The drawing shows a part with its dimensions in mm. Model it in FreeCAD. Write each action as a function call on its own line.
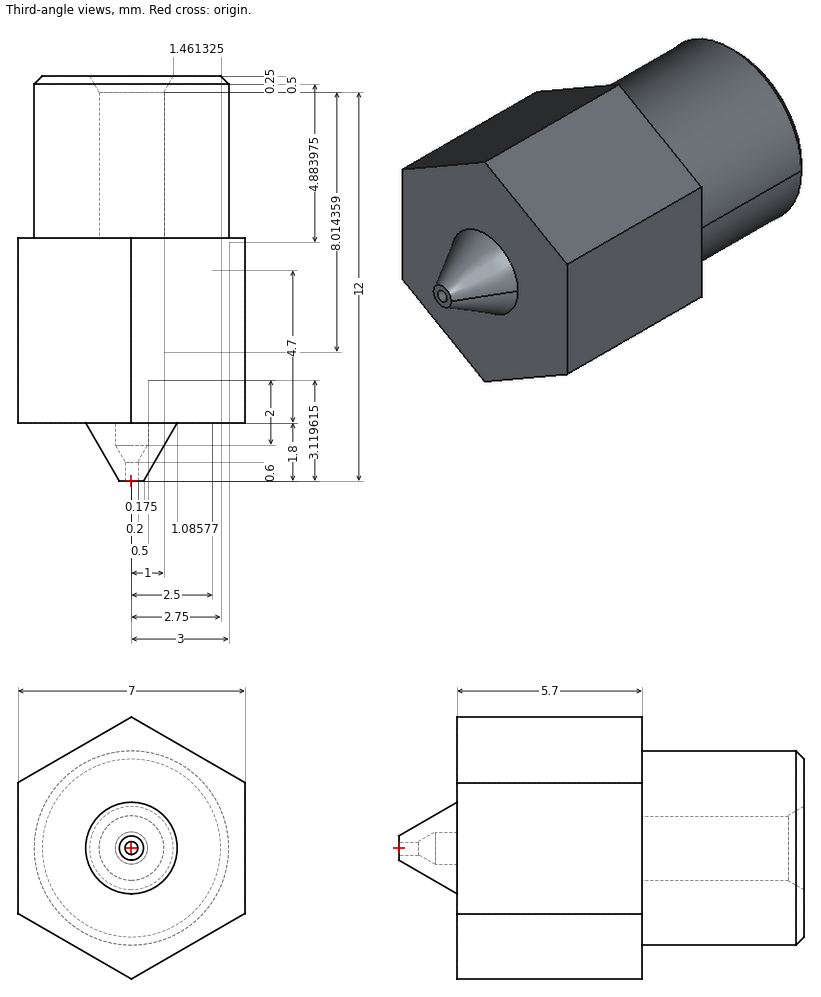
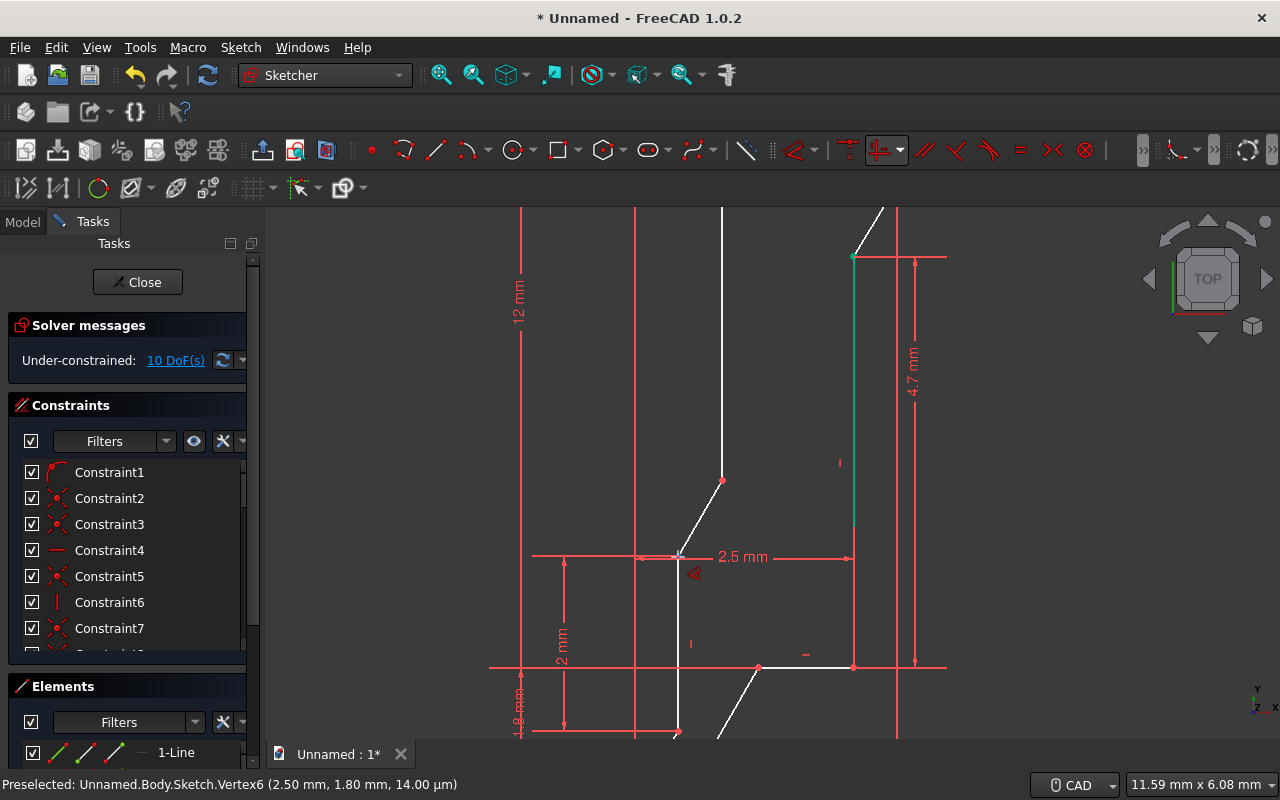
click(678, 556)
click(657, 522)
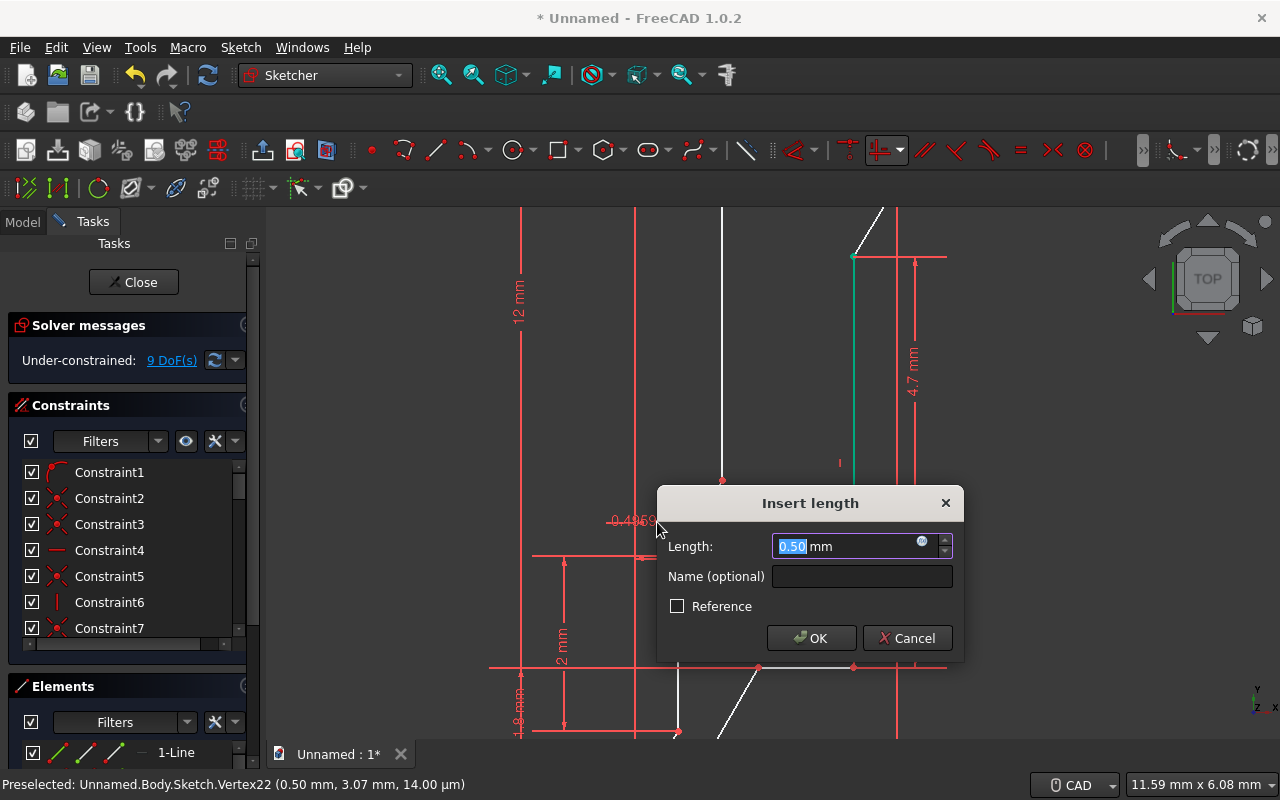
text(0.5)
key(Return)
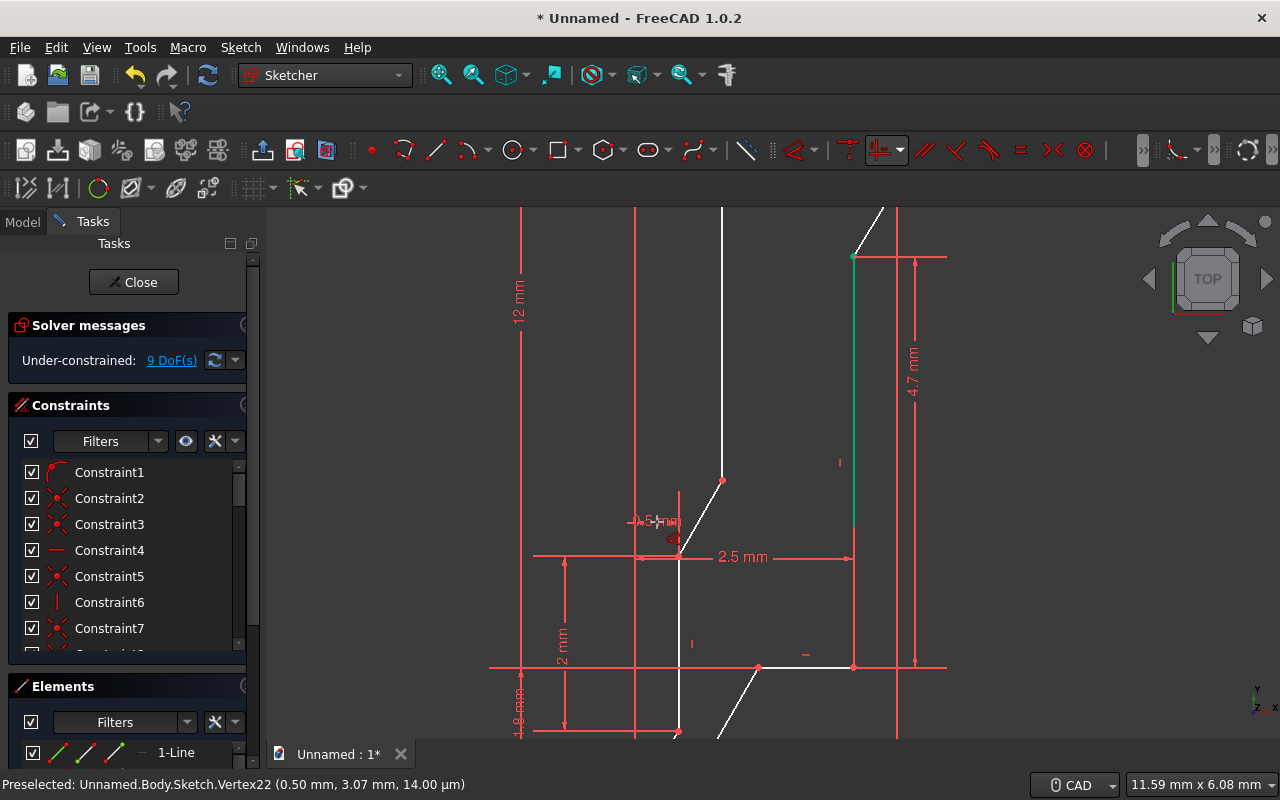
scroll(678, 557, down, 6)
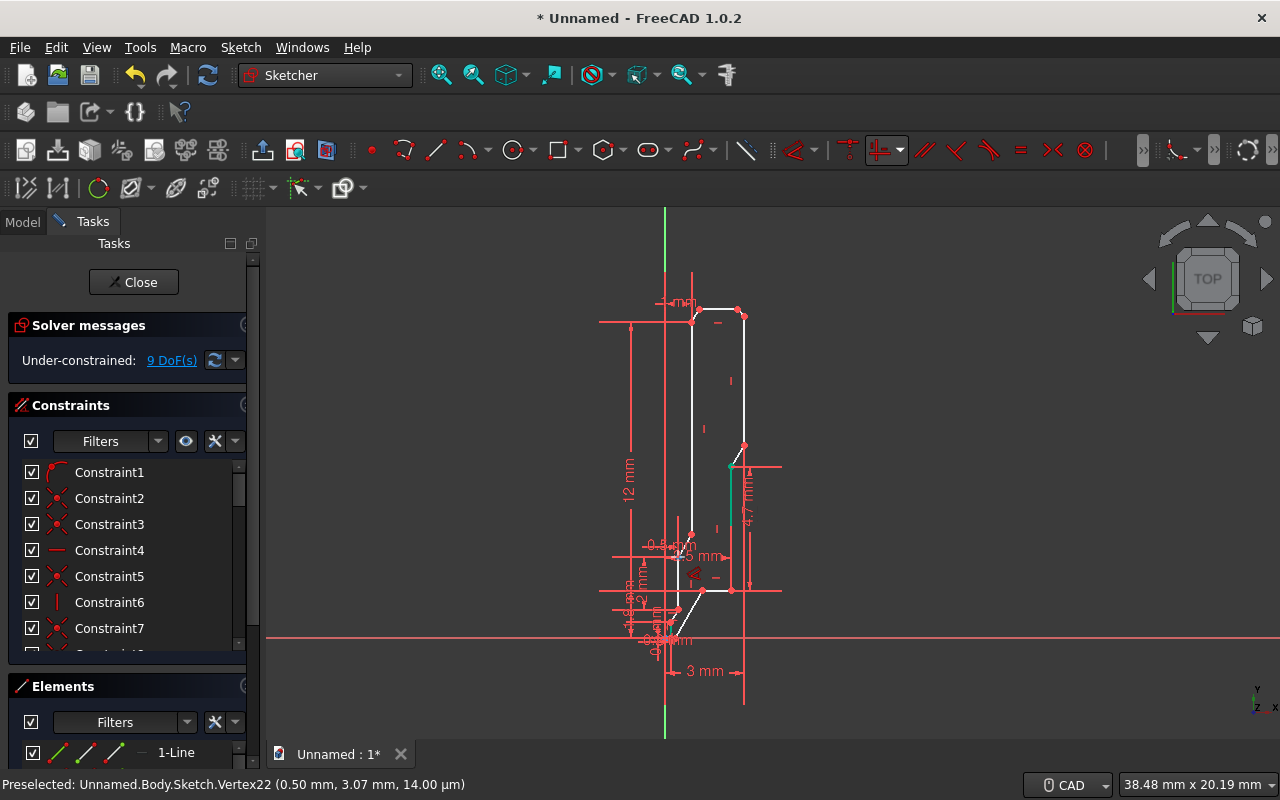
scroll(697, 313, up, 6)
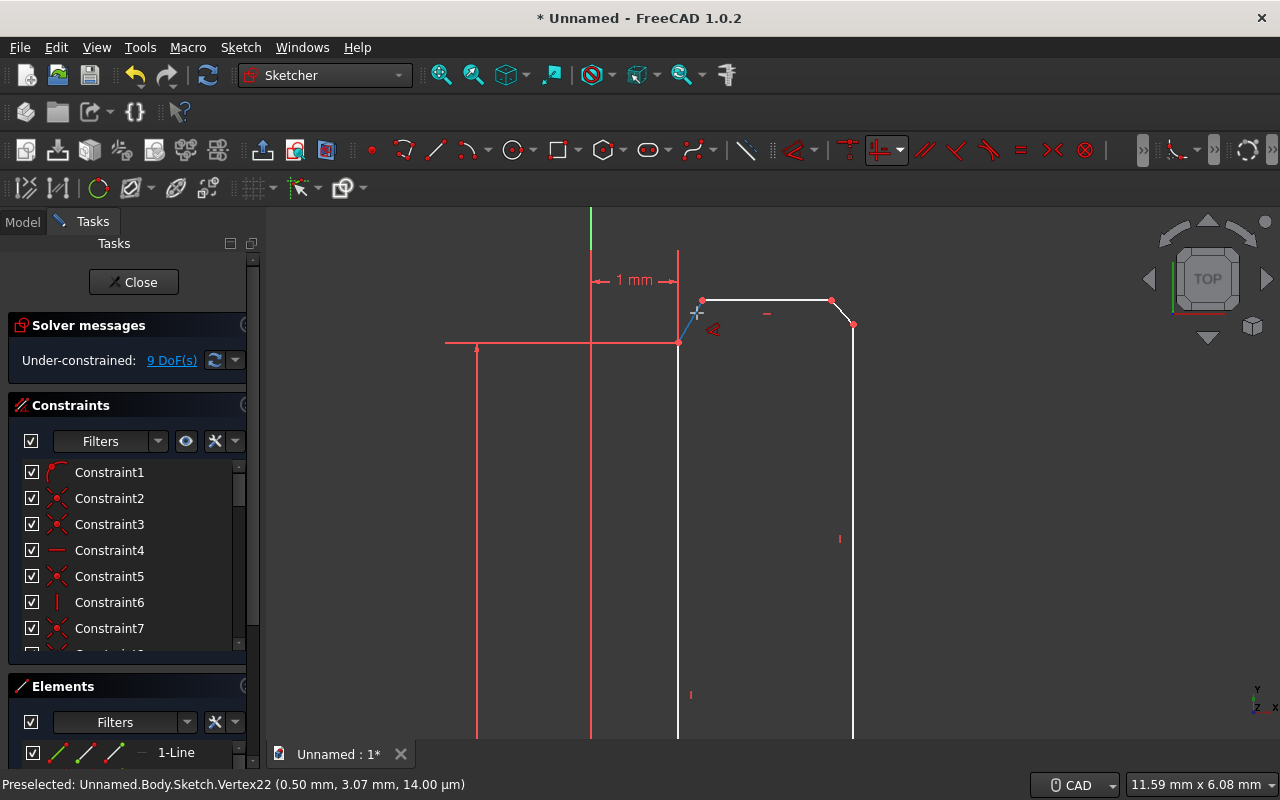
click(695, 313)
click(644, 322)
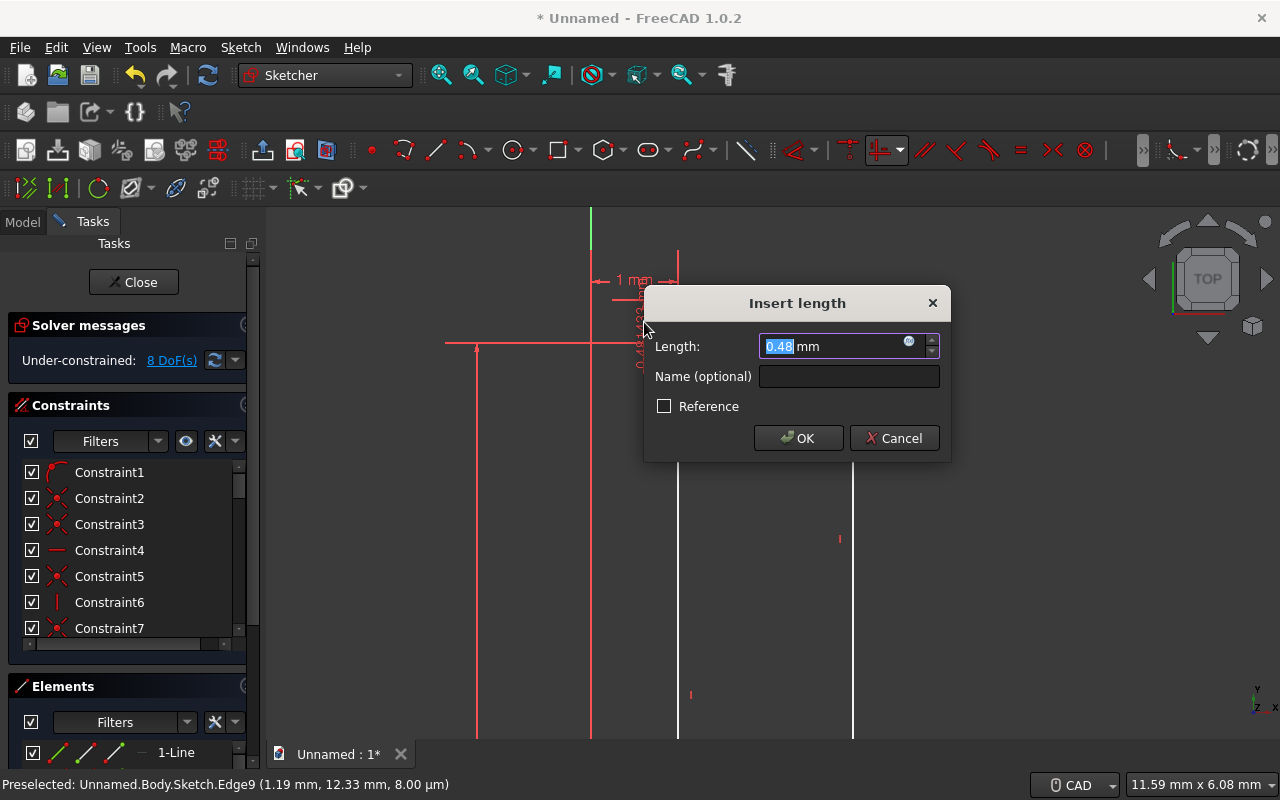
text(0.5)
key(Return)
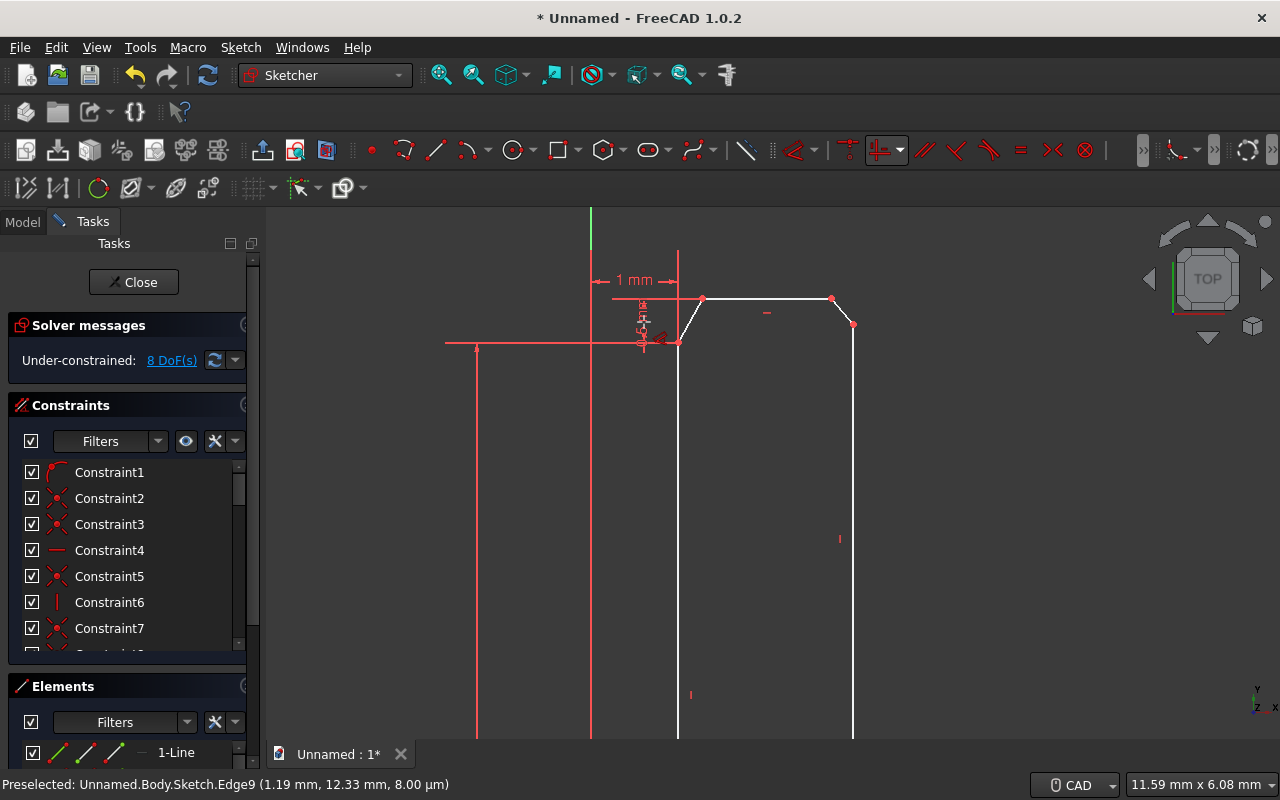
scroll(697, 312, down, 6)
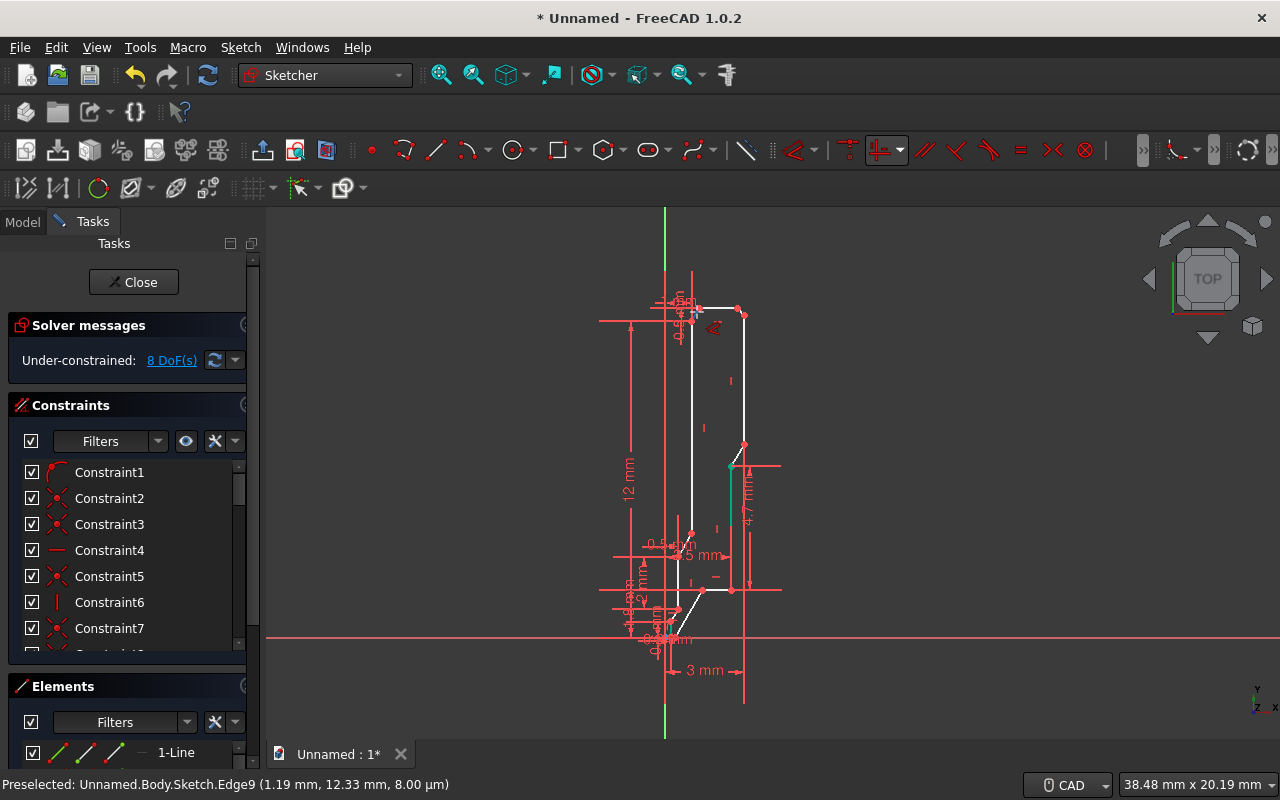
scroll(673, 638, up, 11)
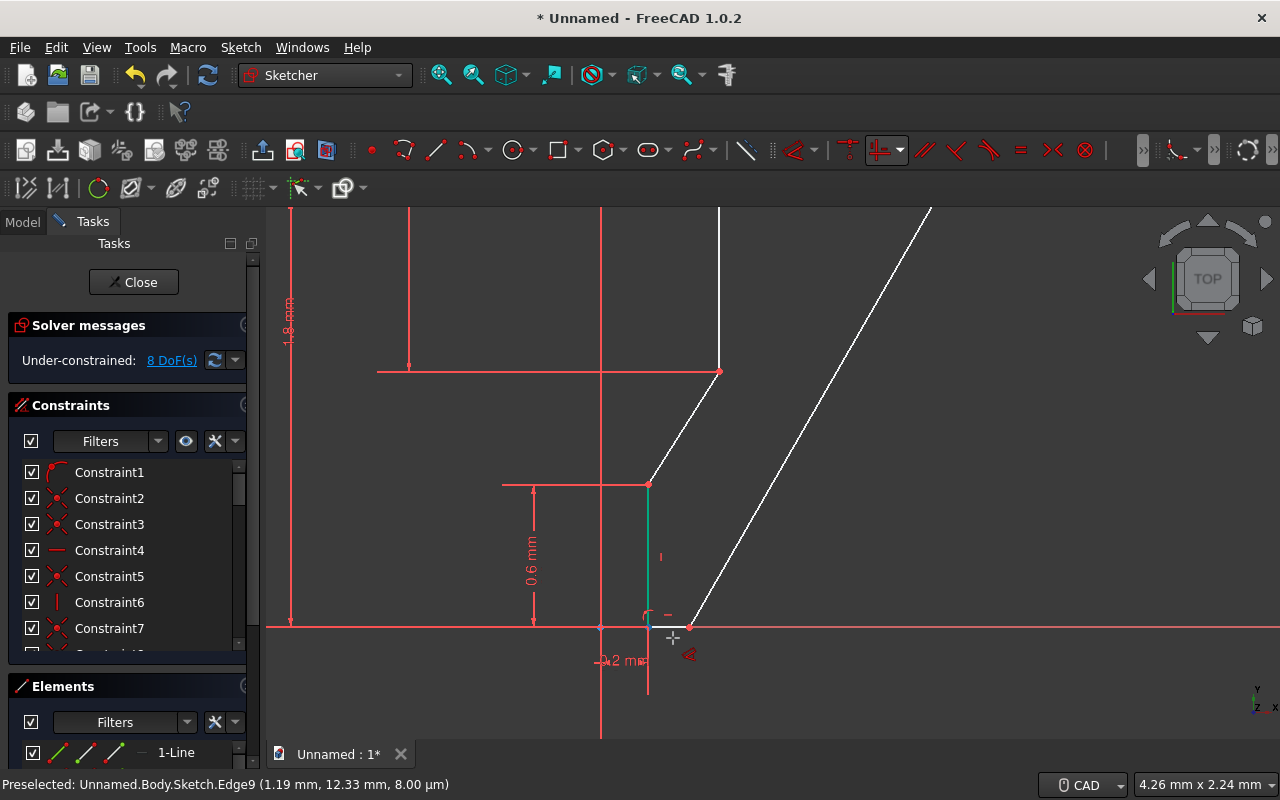
click(669, 627)
click(669, 593)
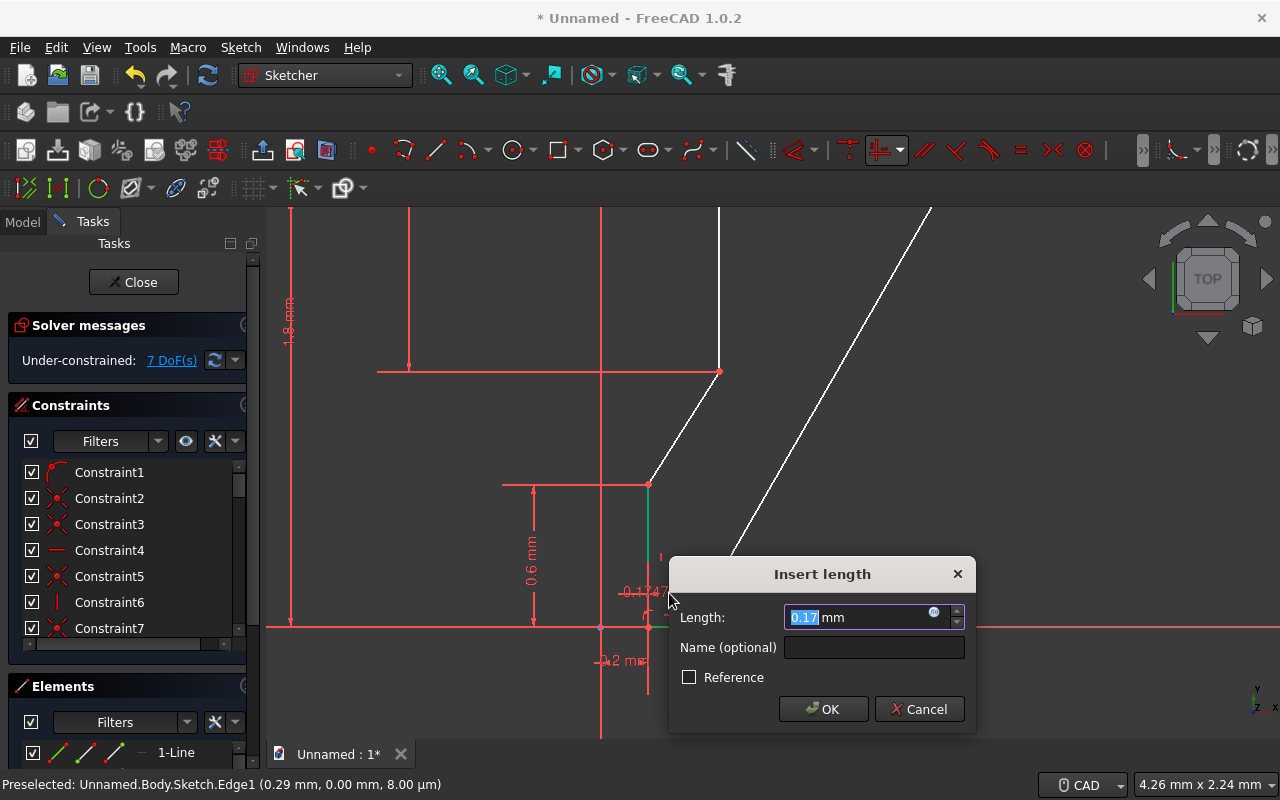
text(0.175)
key(Return)